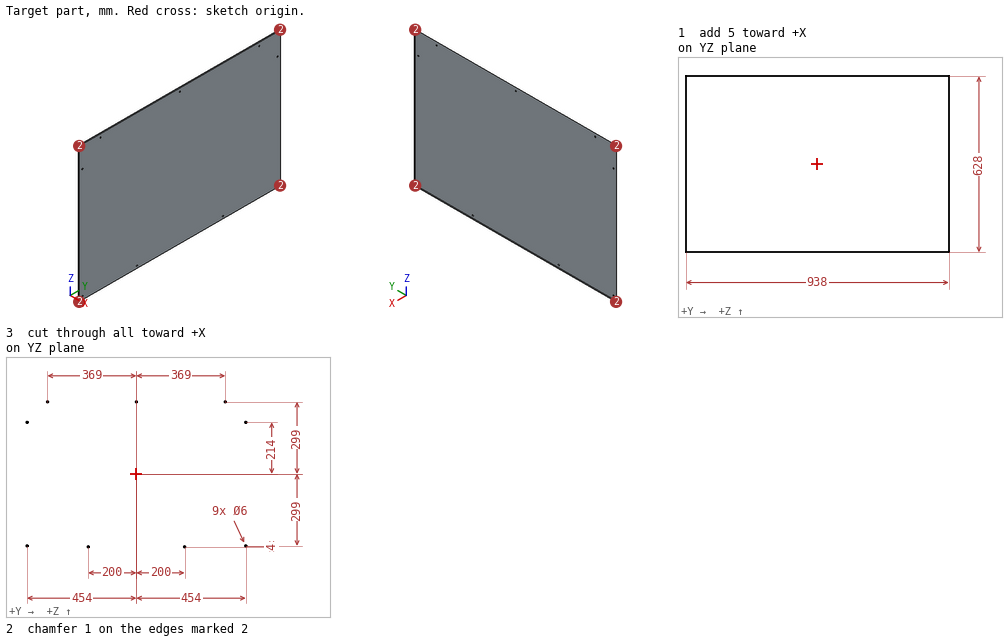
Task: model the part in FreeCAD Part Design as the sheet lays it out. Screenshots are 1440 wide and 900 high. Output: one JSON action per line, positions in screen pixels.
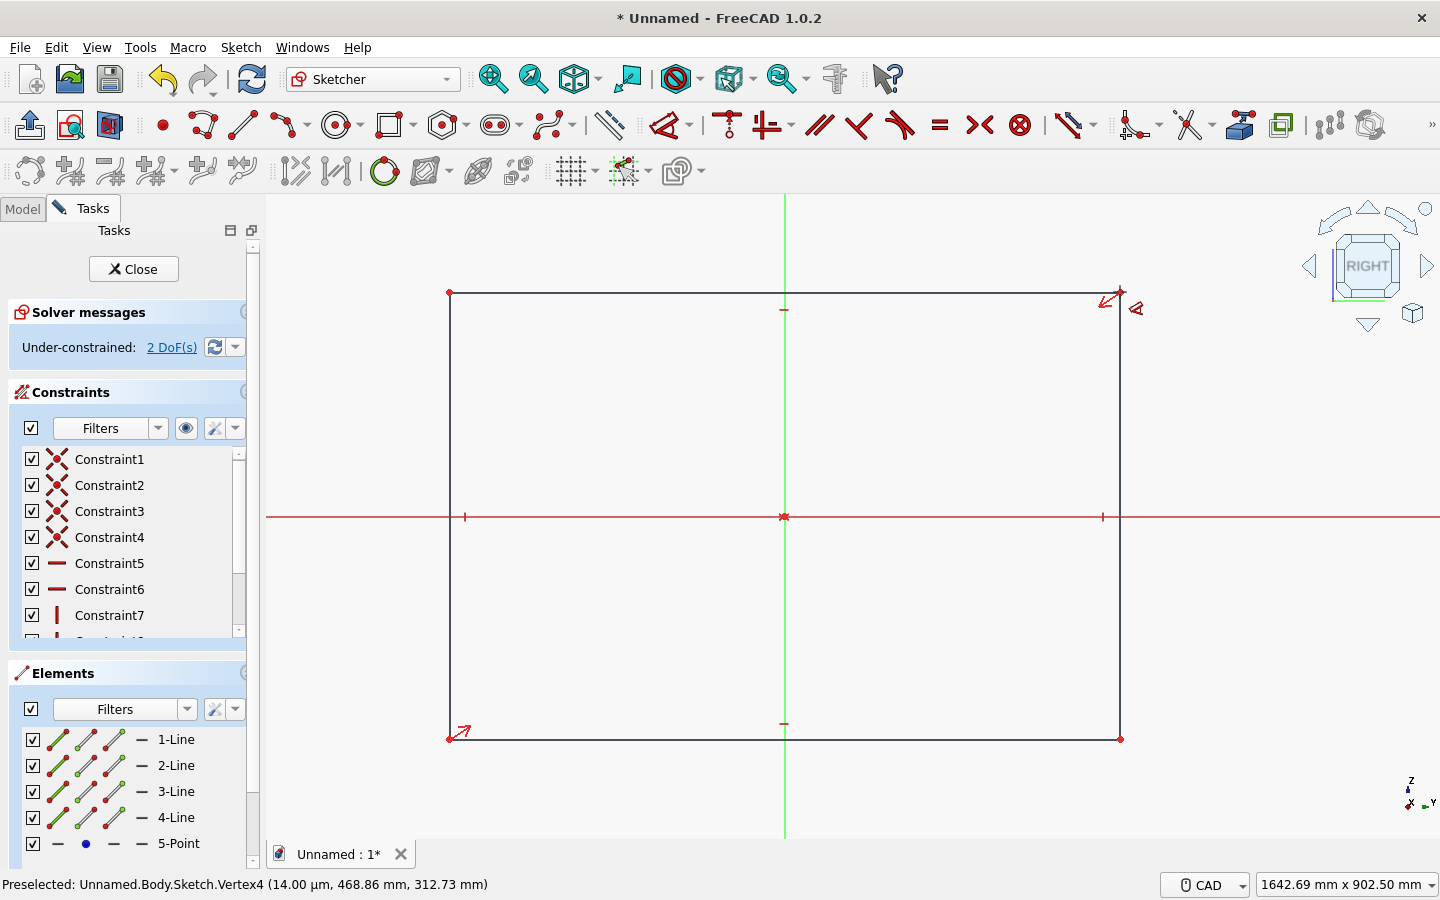
{"action": "left_click", "coordinate": [651, 740]}
{"action": "left_click", "coordinate": [631, 774]}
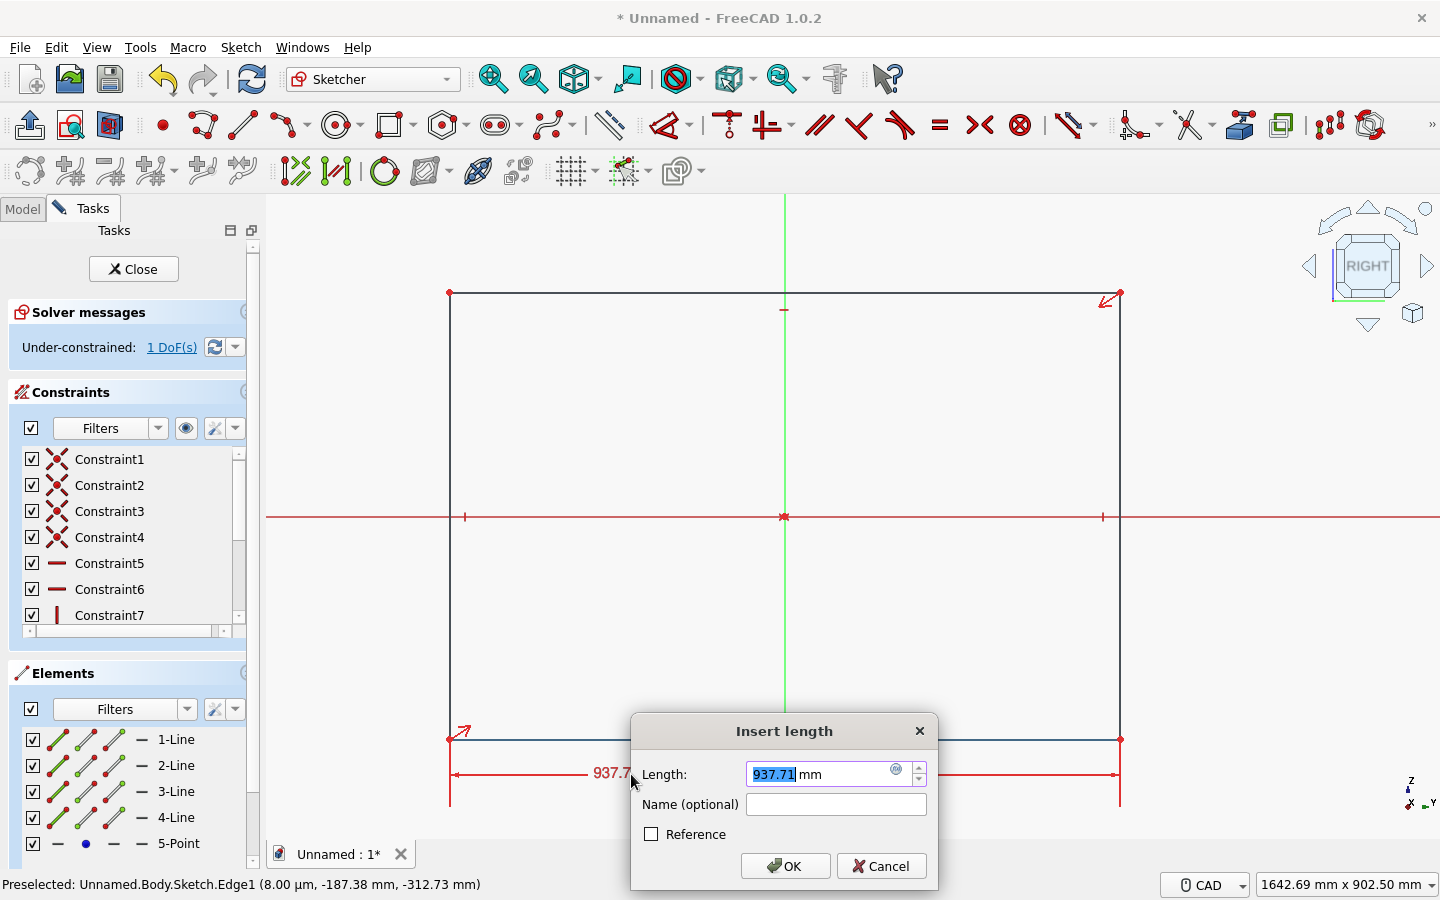
{"action": "type", "text": "938"}
{"action": "key", "text": "Return"}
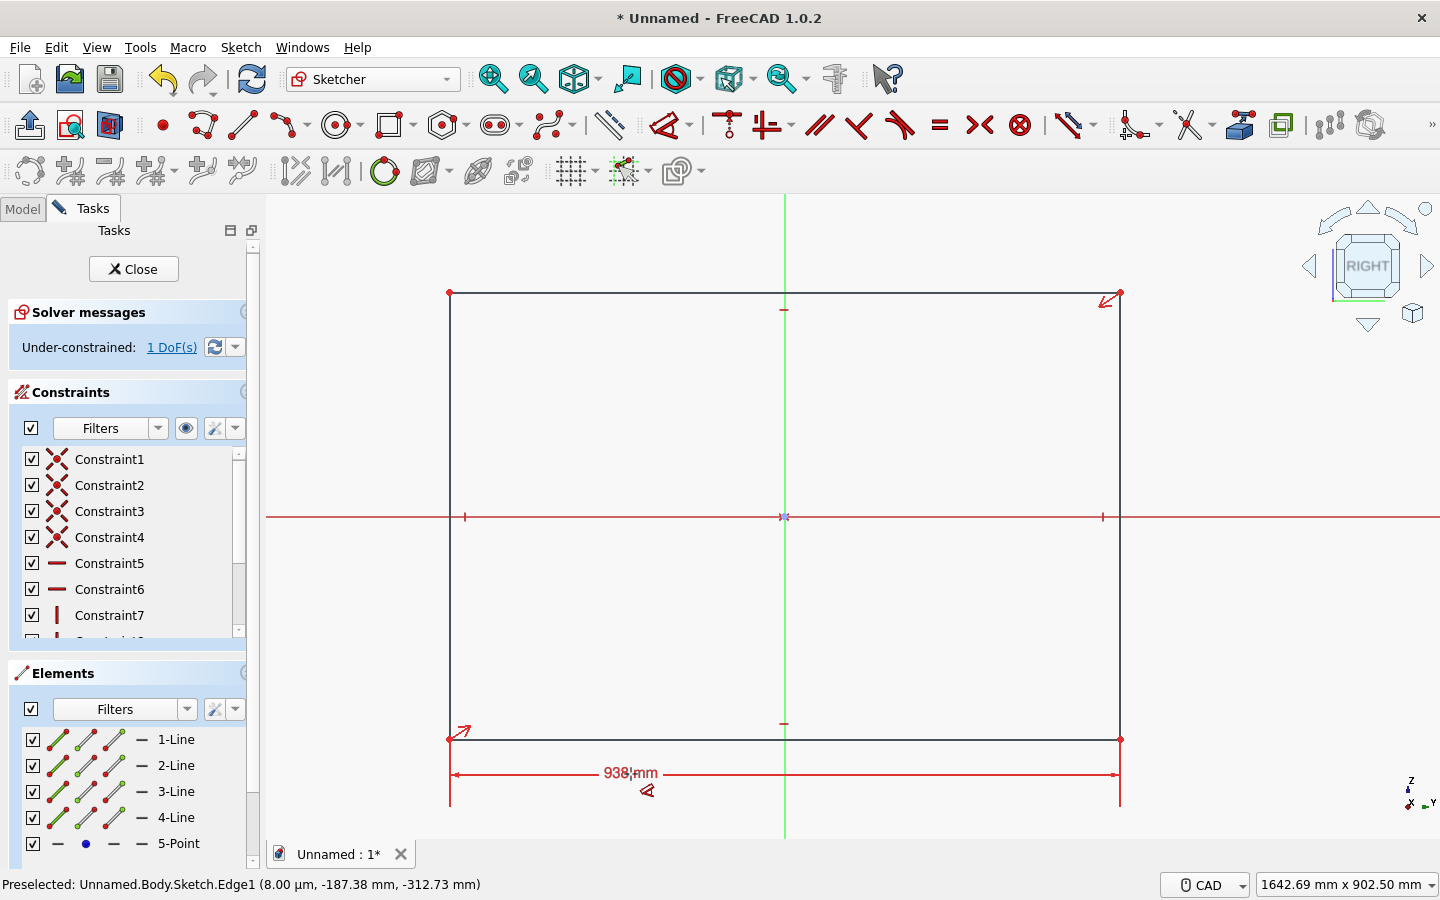
{"action": "left_click", "coordinate": [1120, 606]}
{"action": "left_click", "coordinate": [1154, 414]}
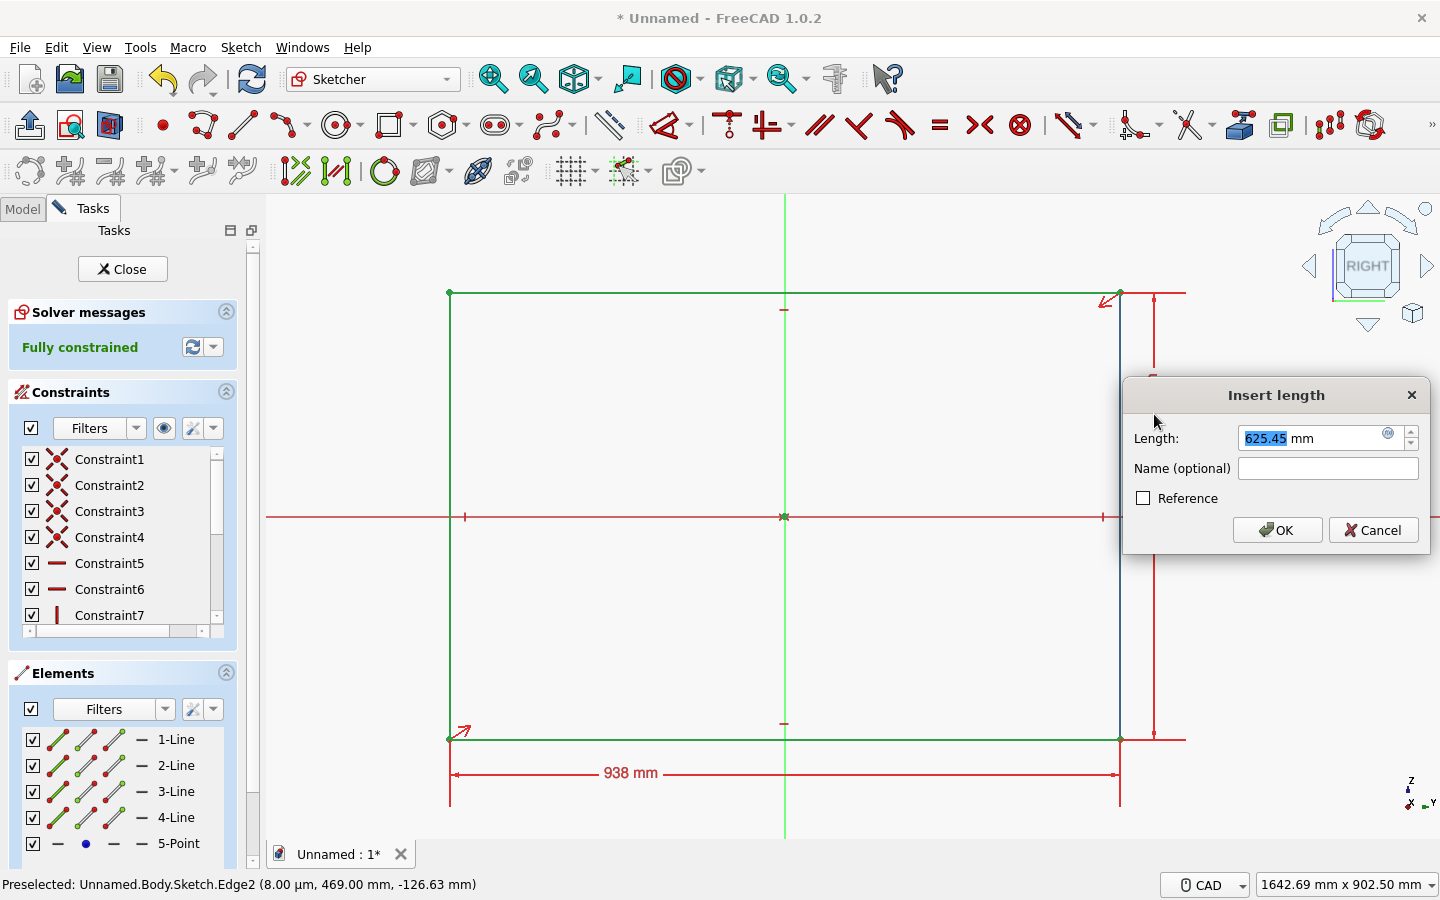
{"action": "type", "text": "628"}
{"action": "key", "text": "Return"}
{"action": "key", "text": "Escape"}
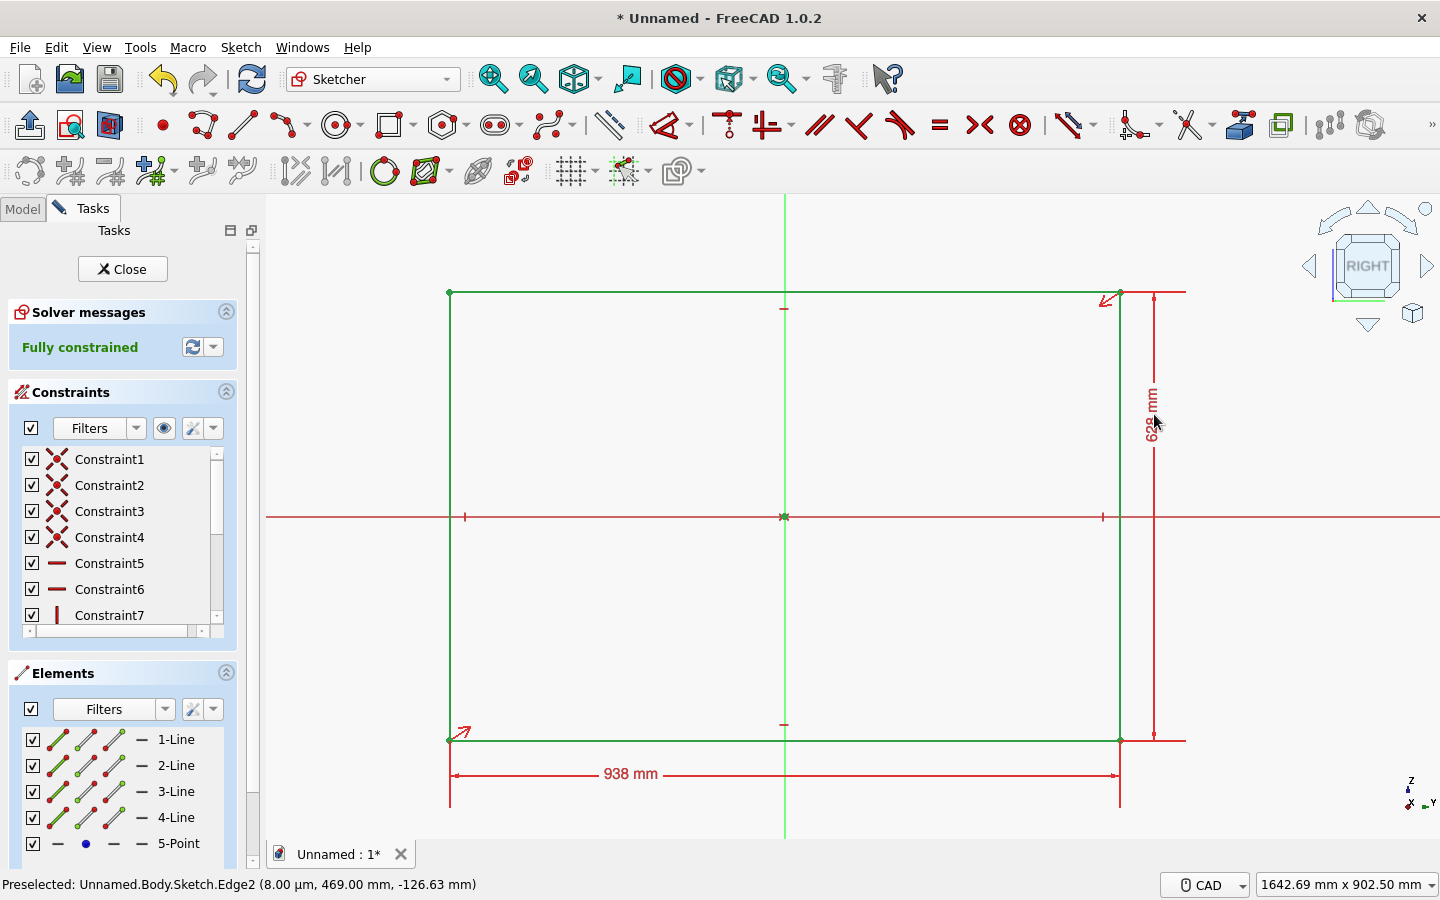
{"action": "left_click", "coordinate": [123, 269]}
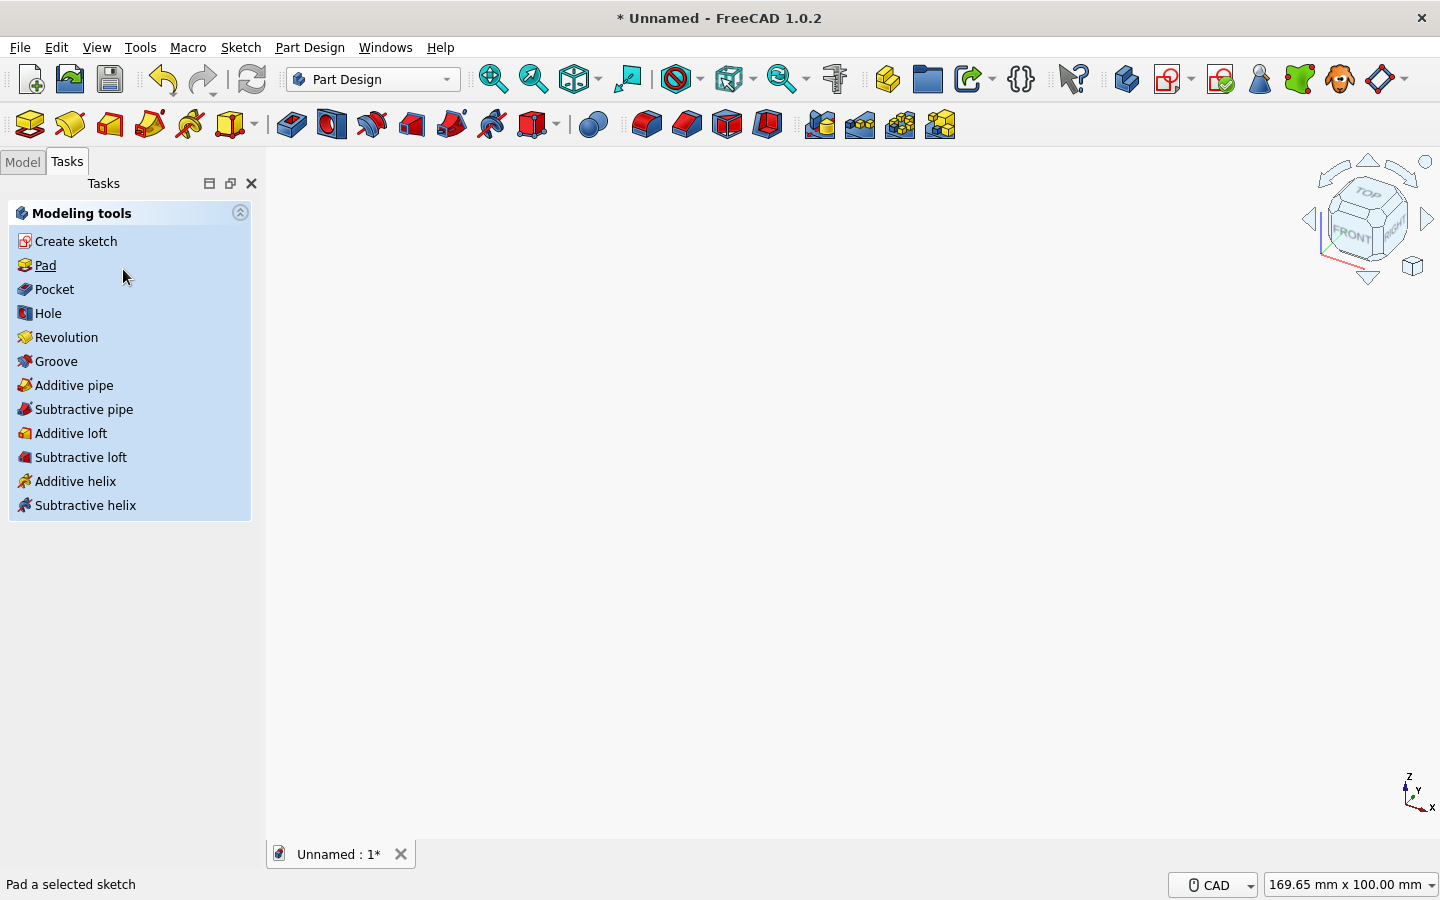
{"action": "left_click", "coordinate": [30, 124]}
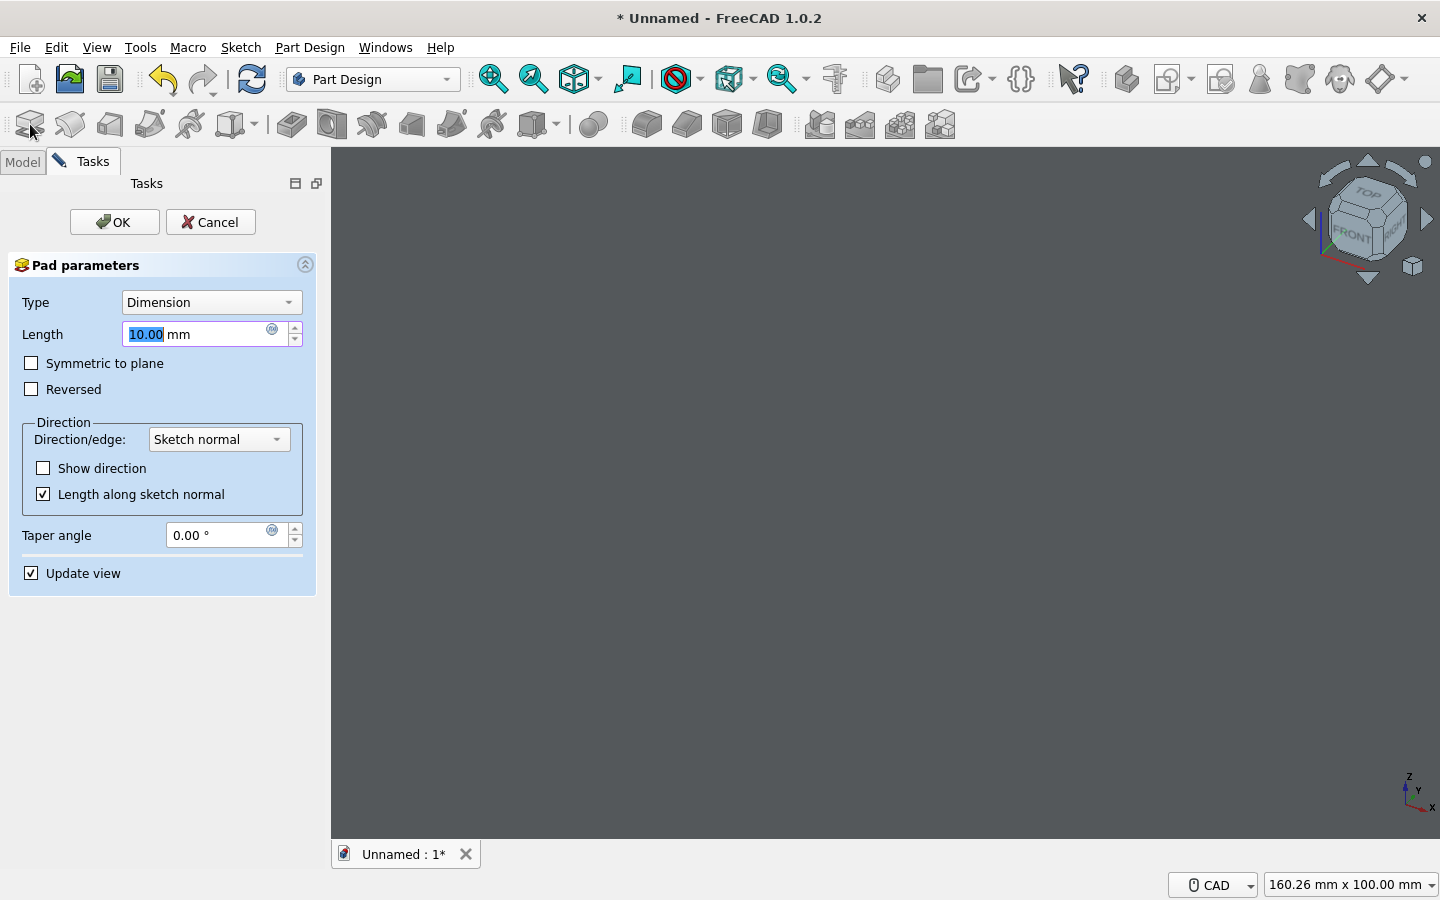
{"action": "type", "text": "5"}
{"action": "key", "text": "Tab"}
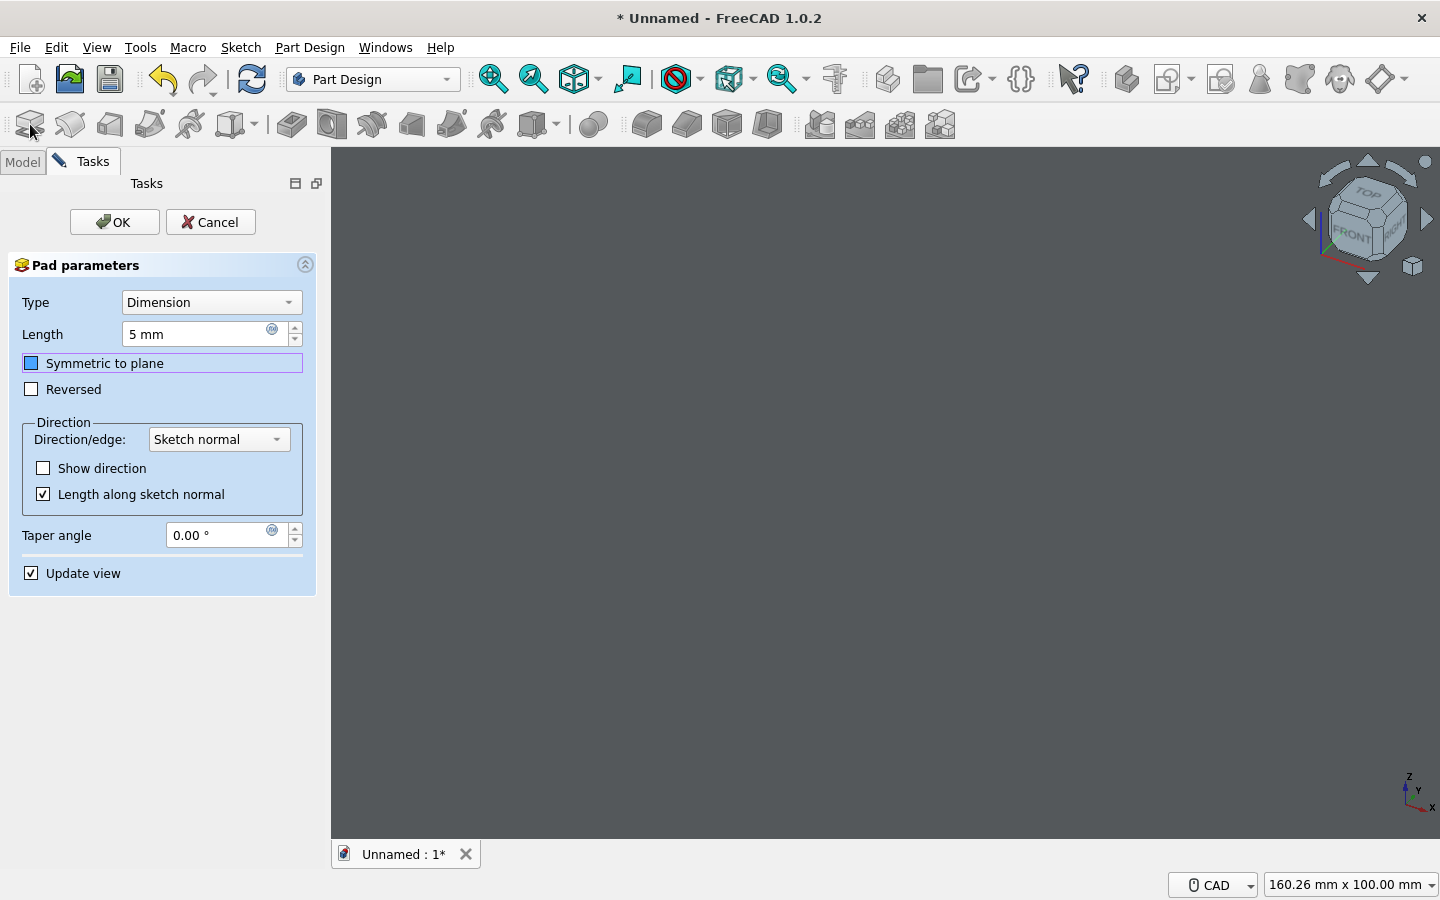
{"action": "left_click", "coordinate": [115, 222]}